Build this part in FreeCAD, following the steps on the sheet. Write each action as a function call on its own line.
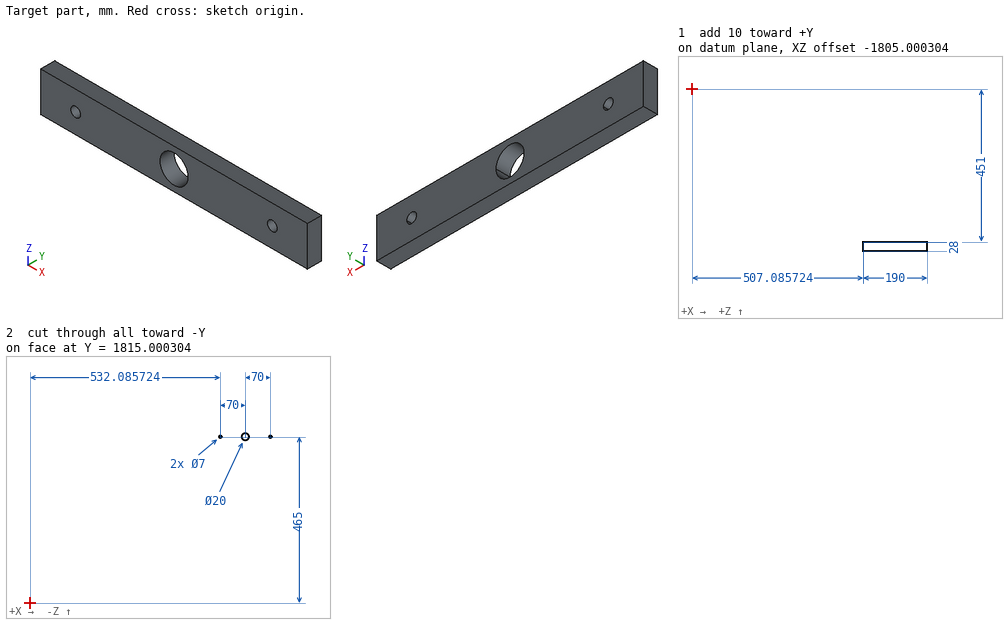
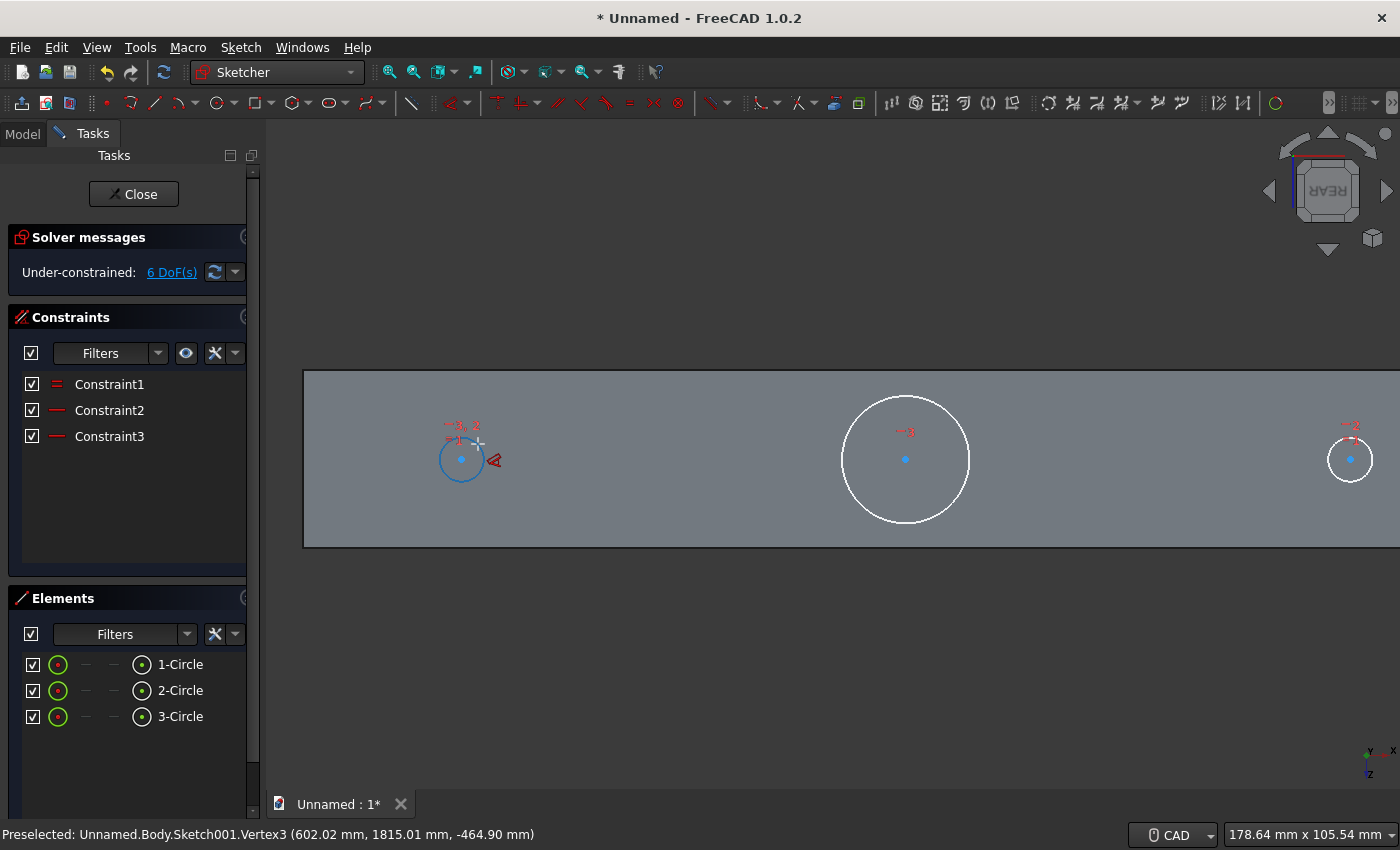
click(477, 444)
click(499, 421)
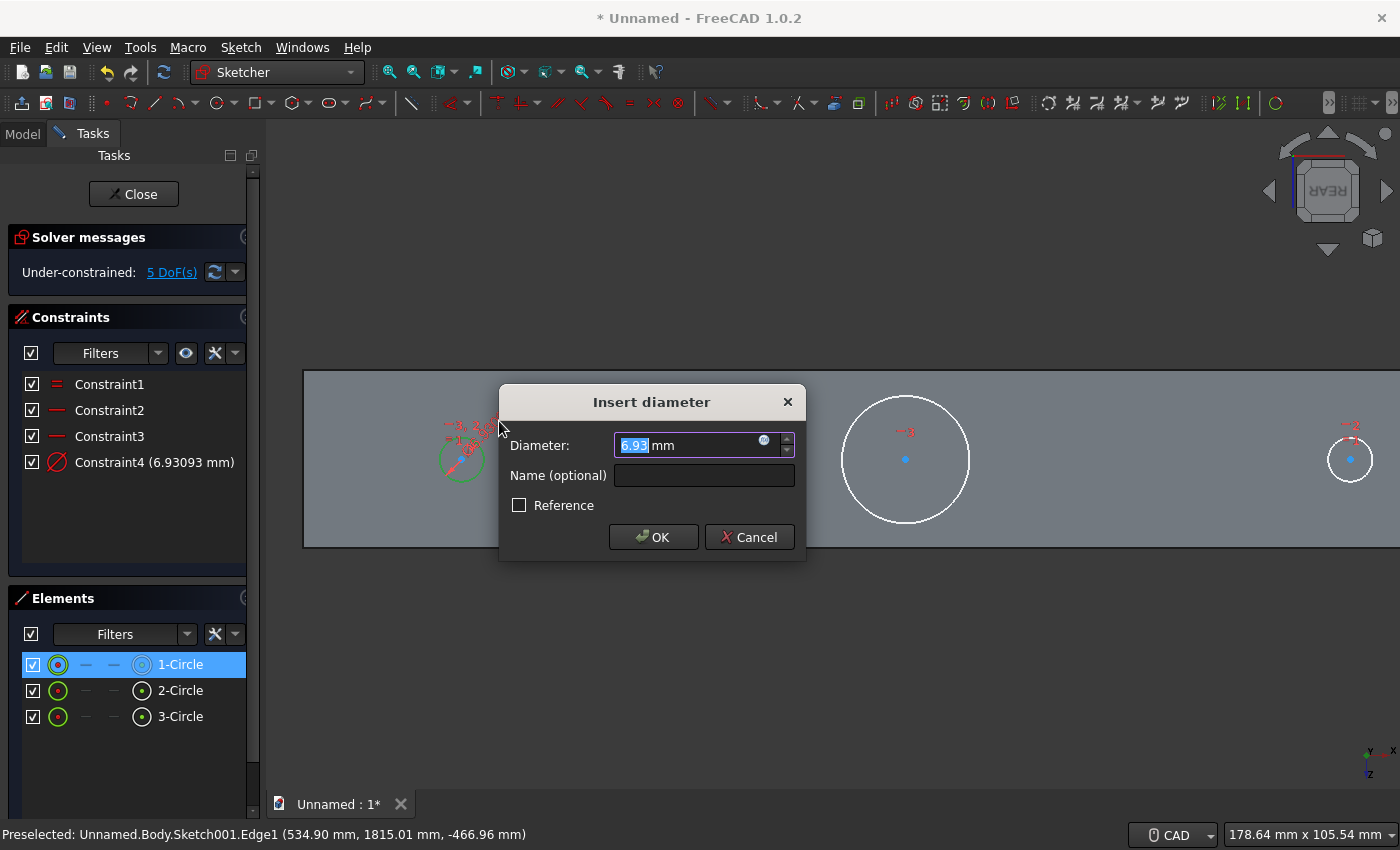
text(7)
key(Return)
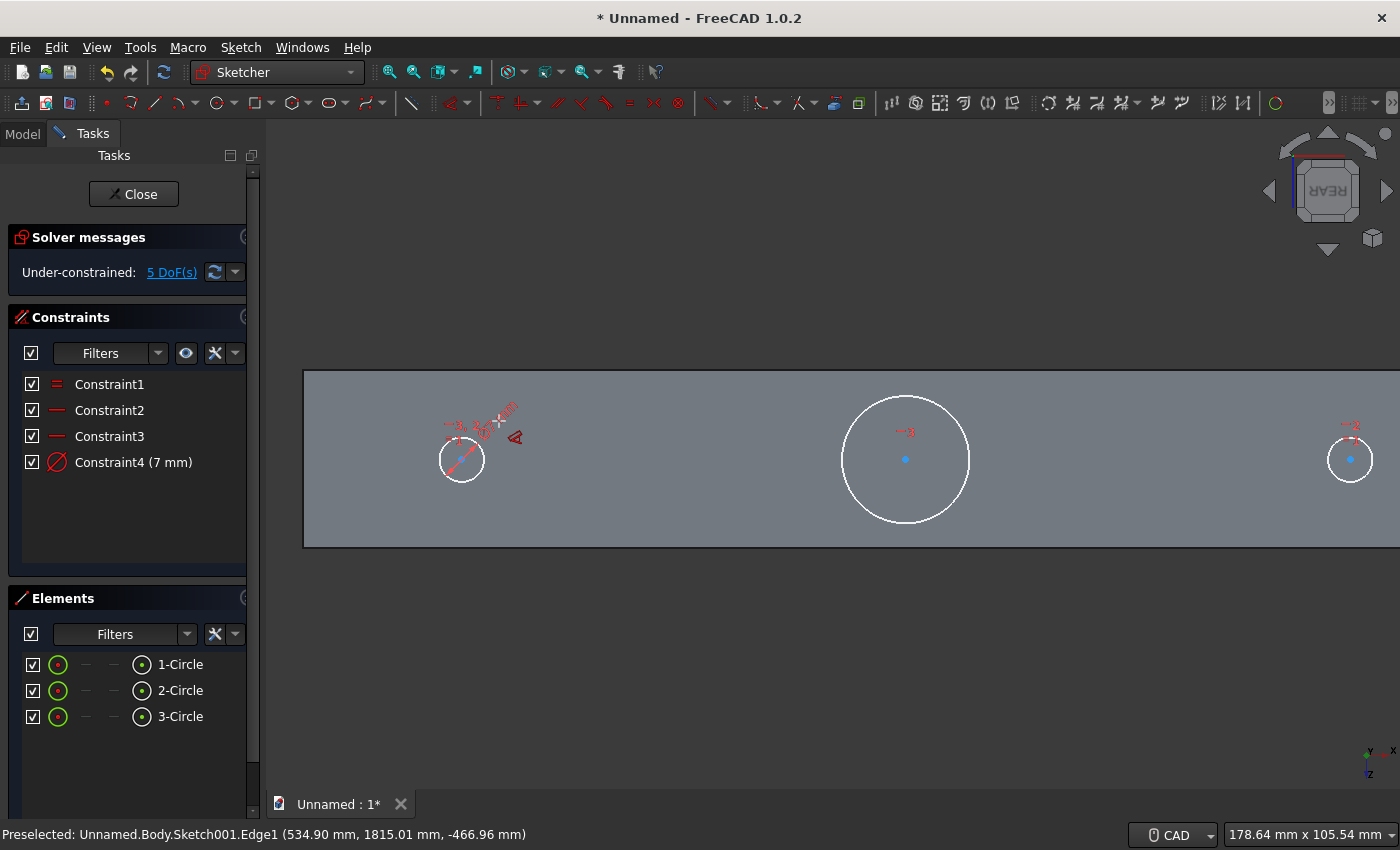
click(951, 415)
click(974, 393)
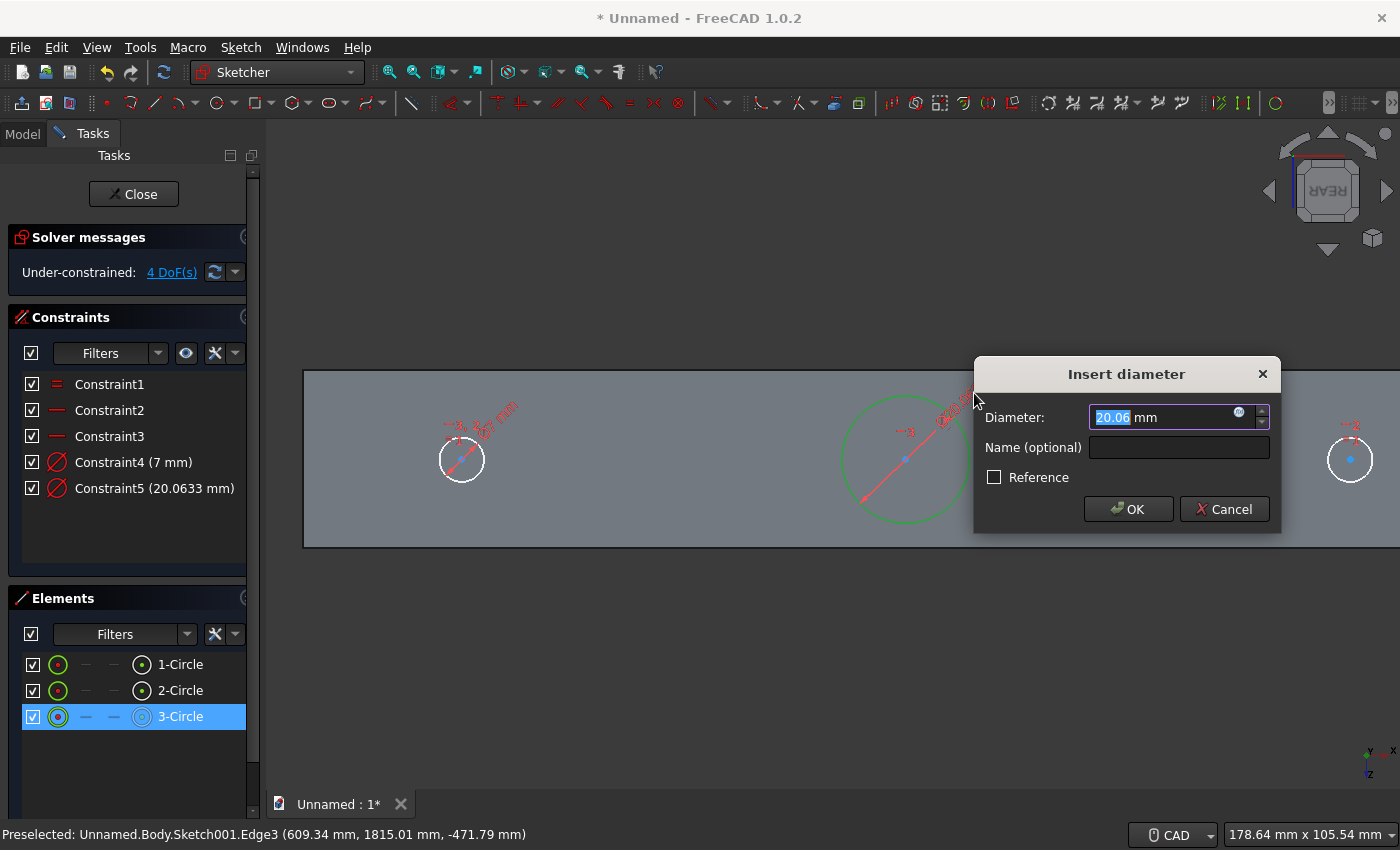
text(20)
key(Return)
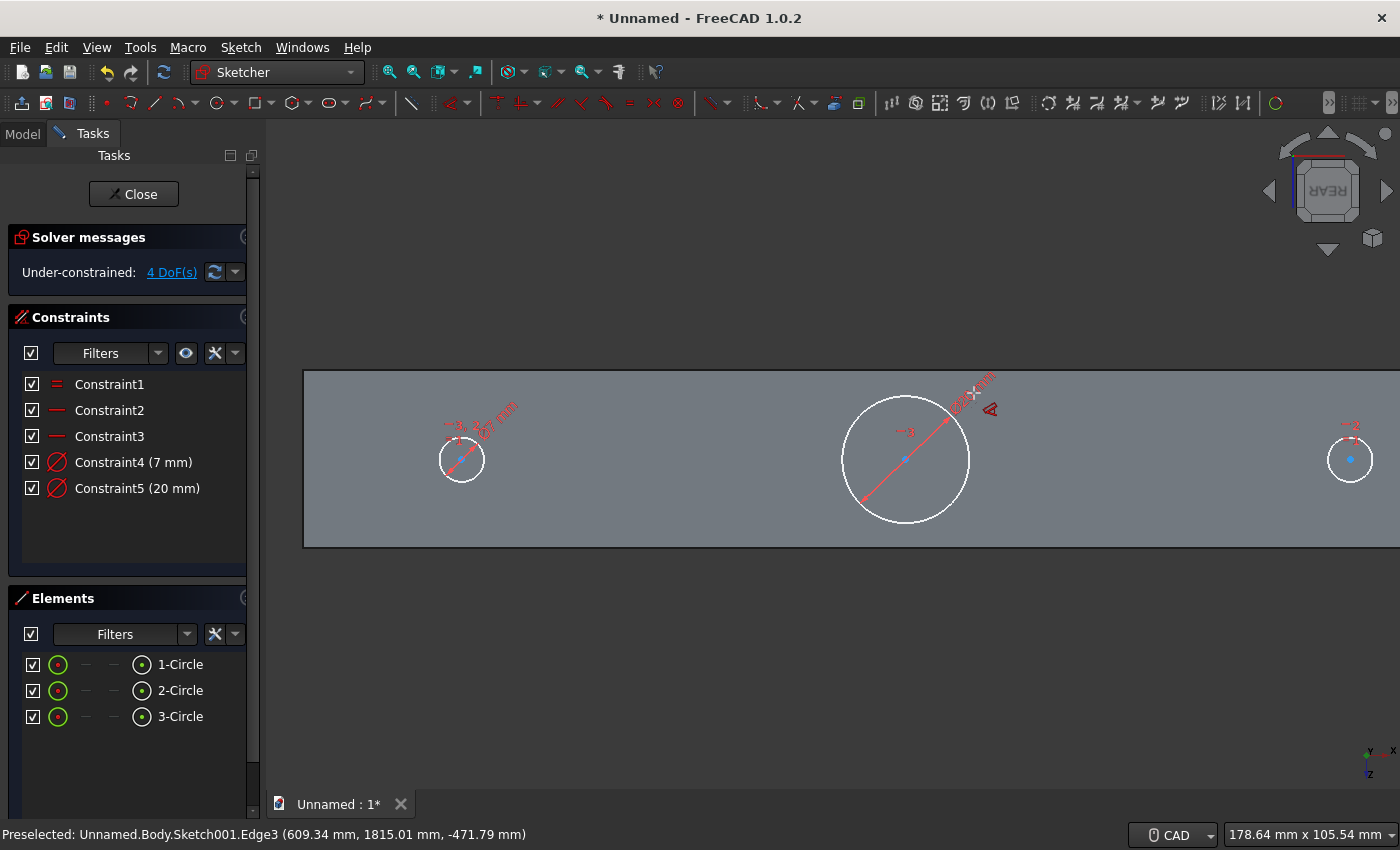
click(462, 460)
click(496, 610)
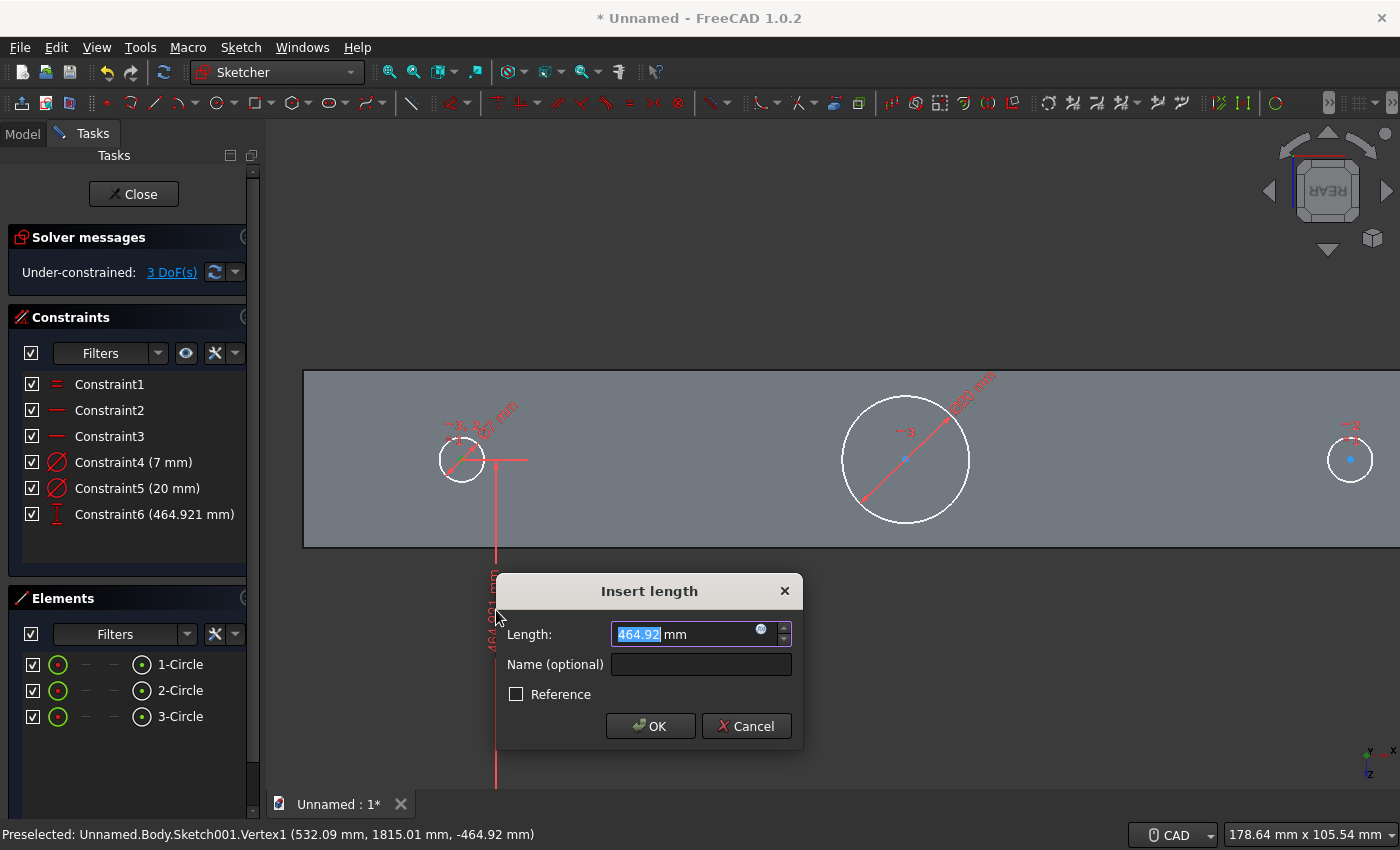
text(465)
key(Return)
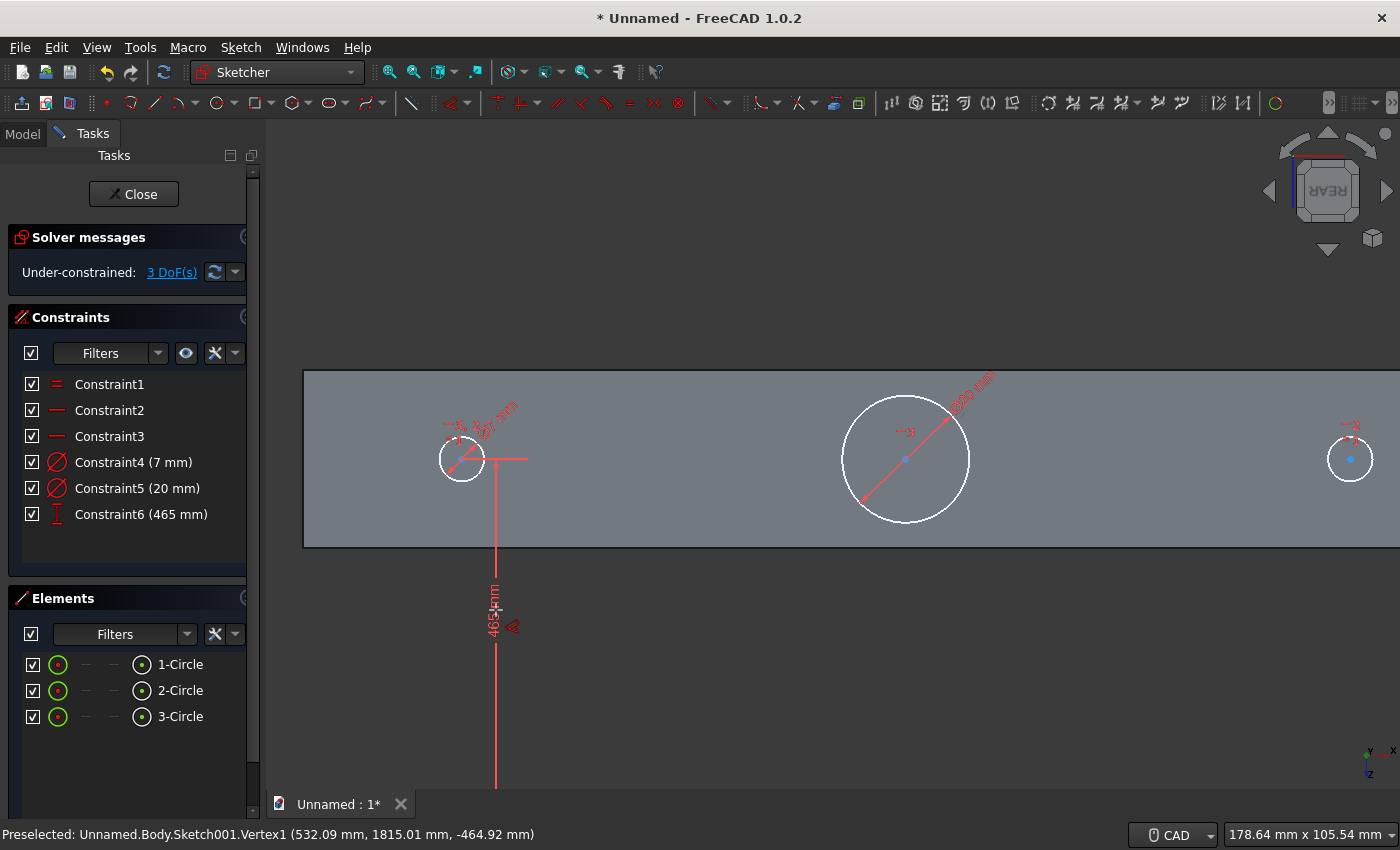
click(462, 459)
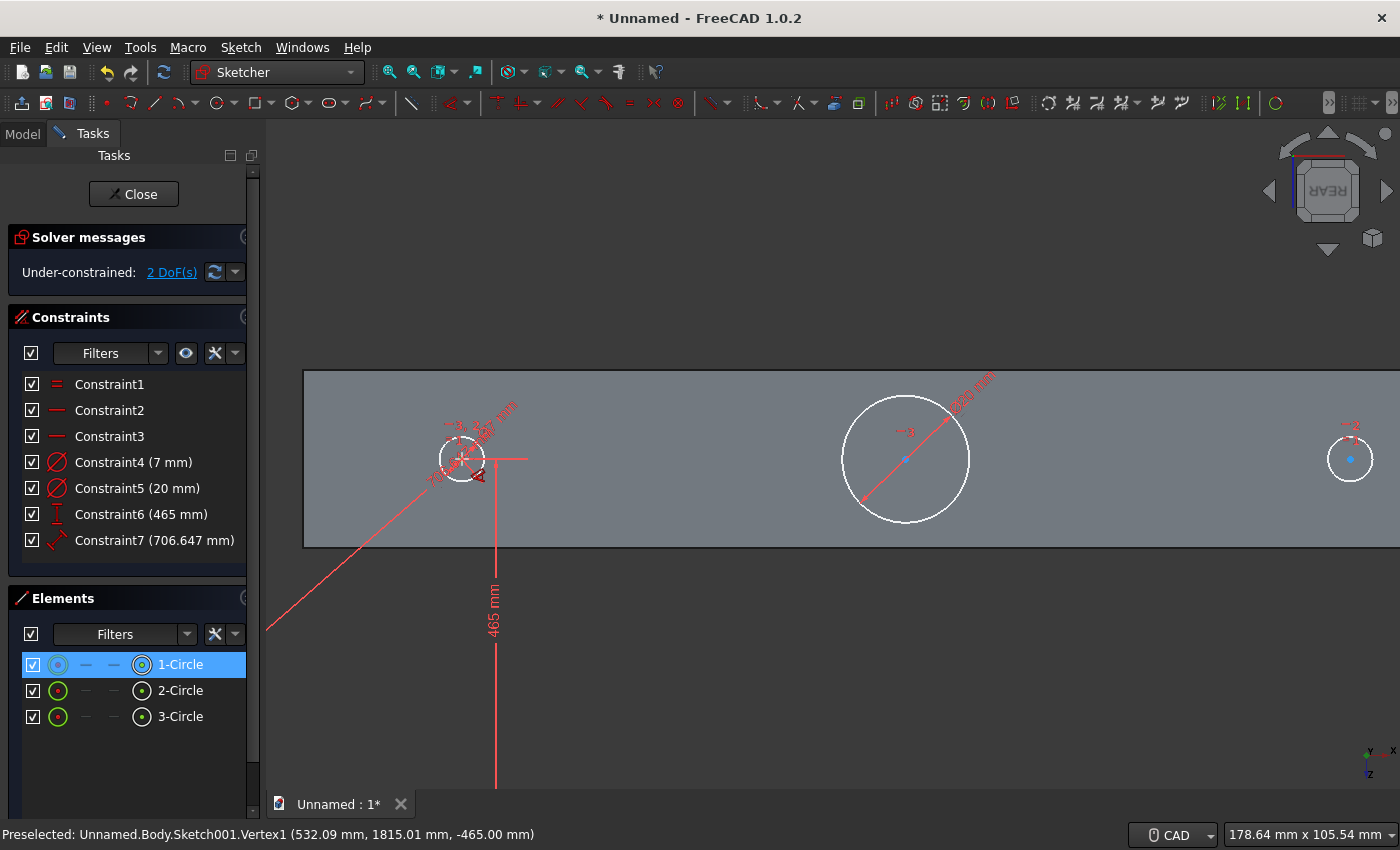
click(906, 459)
click(684, 493)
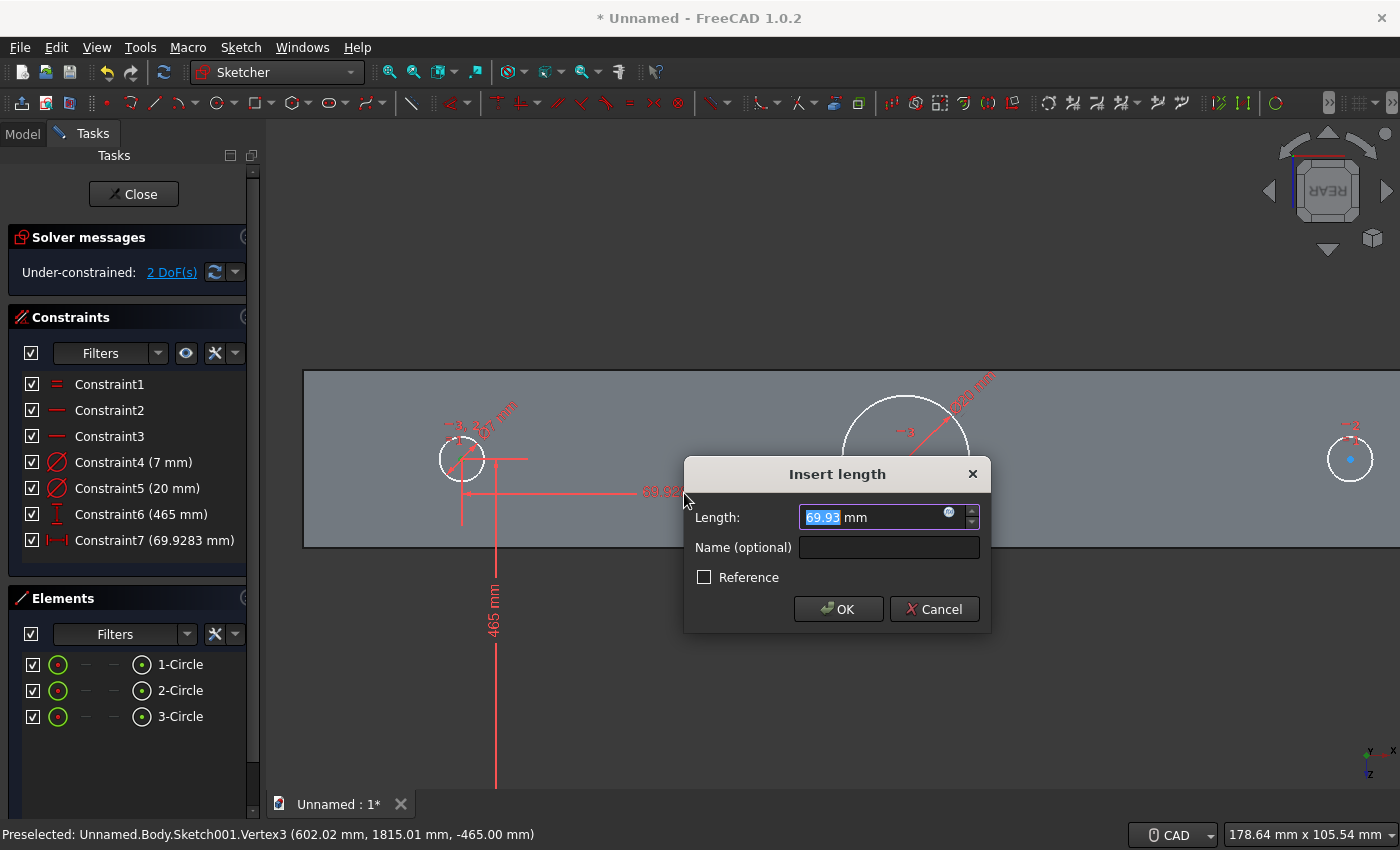
text(70)
key(Return)